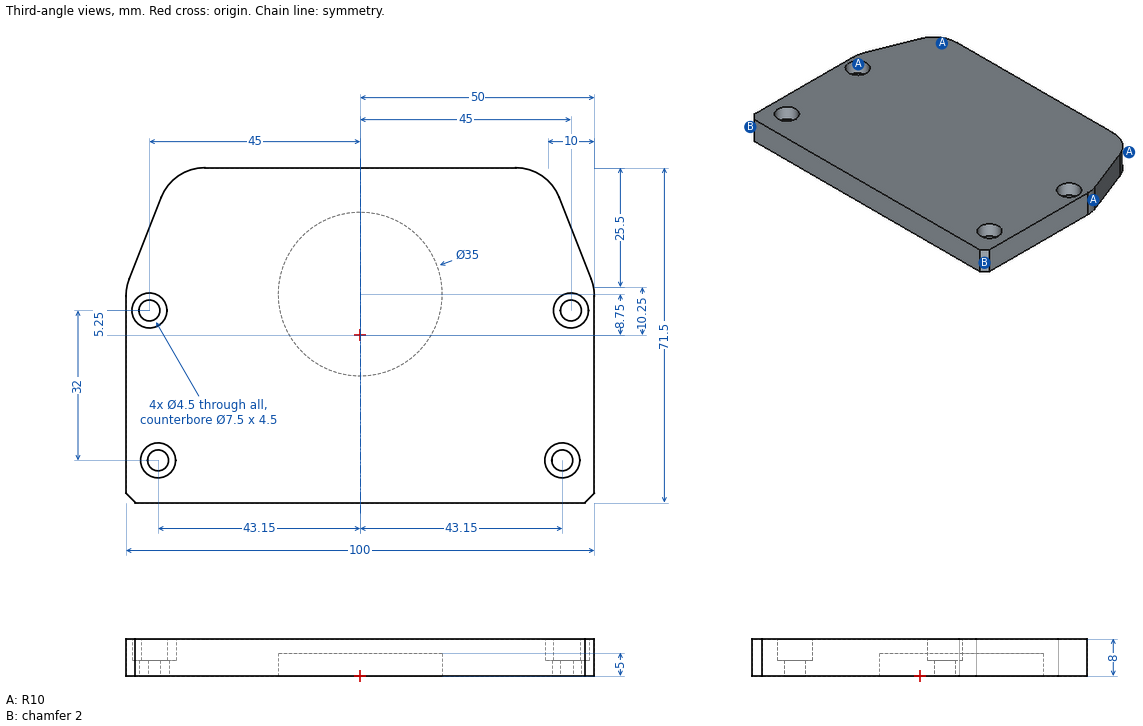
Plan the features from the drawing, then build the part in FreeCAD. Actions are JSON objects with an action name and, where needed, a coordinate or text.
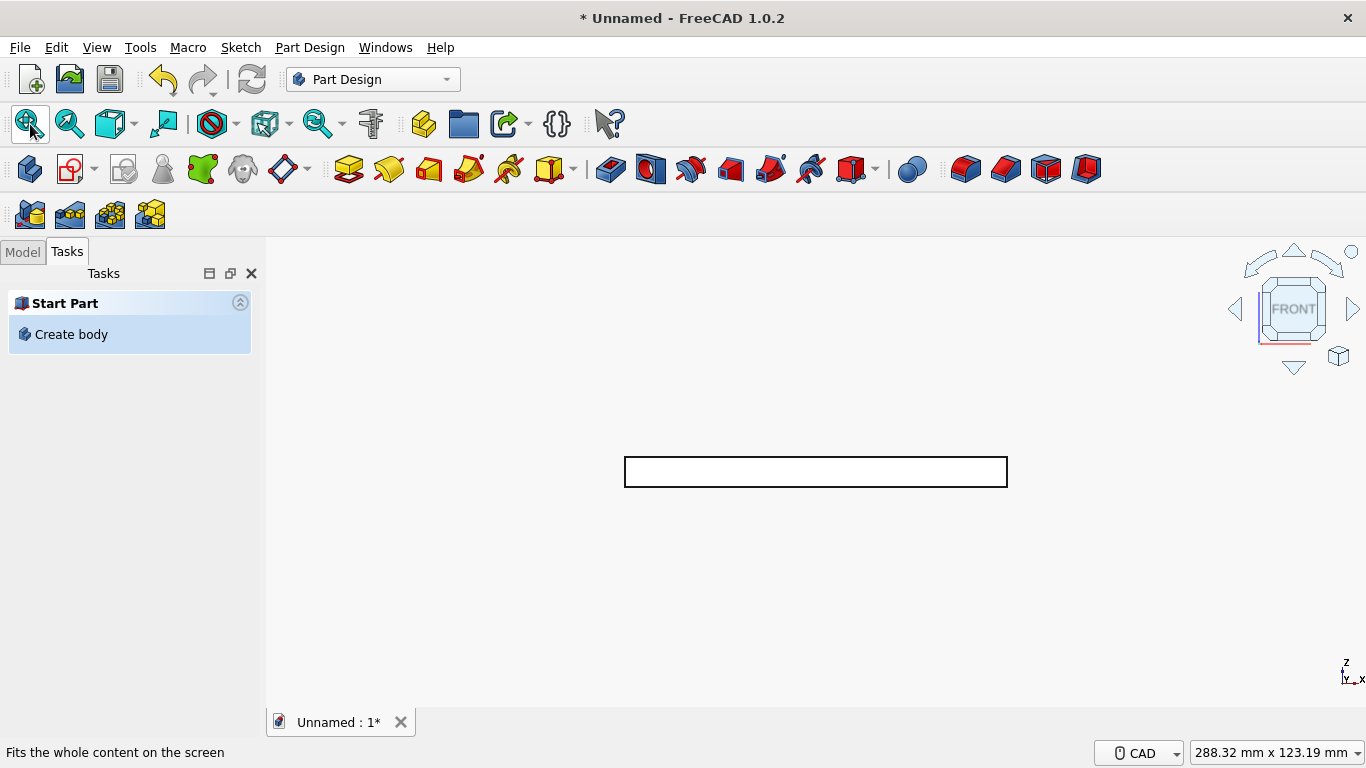
{"action": "key", "text": "3"}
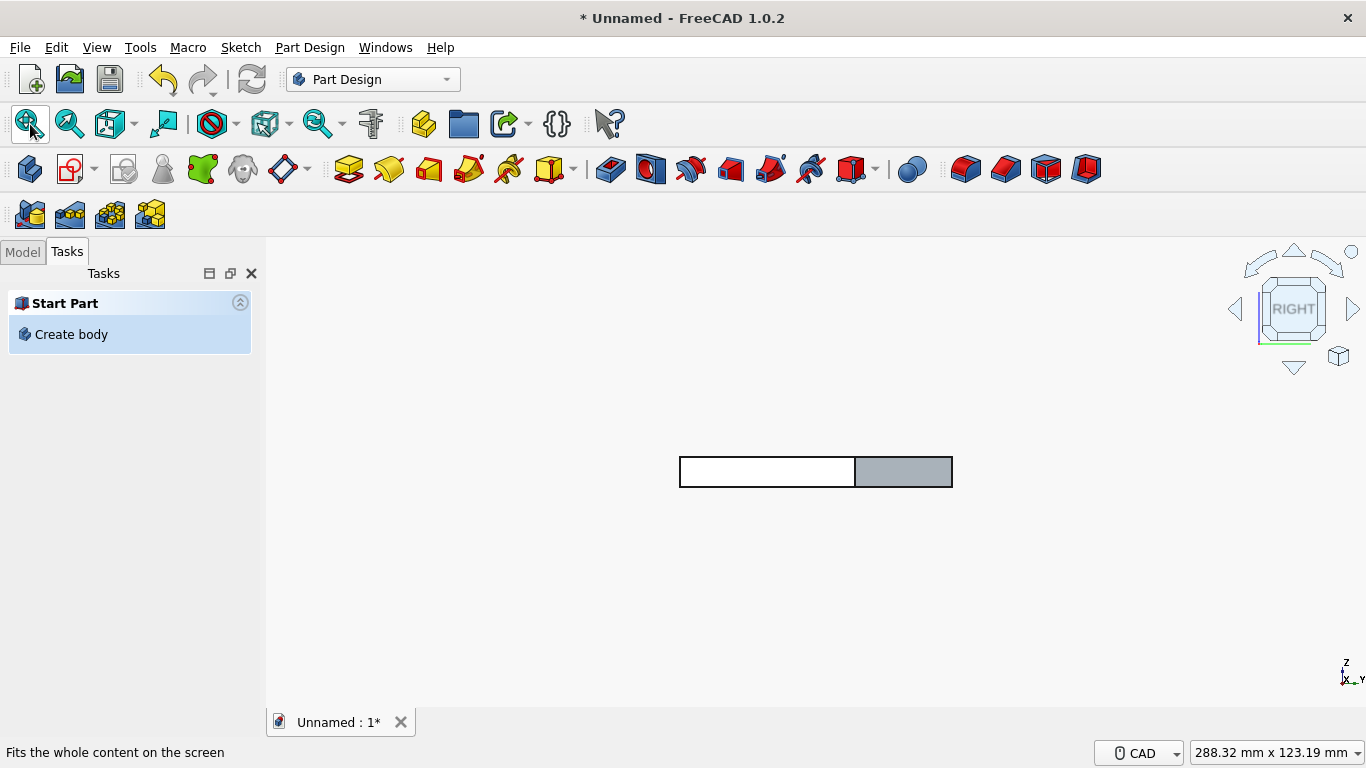
{"action": "left_click", "coordinate": [30, 124]}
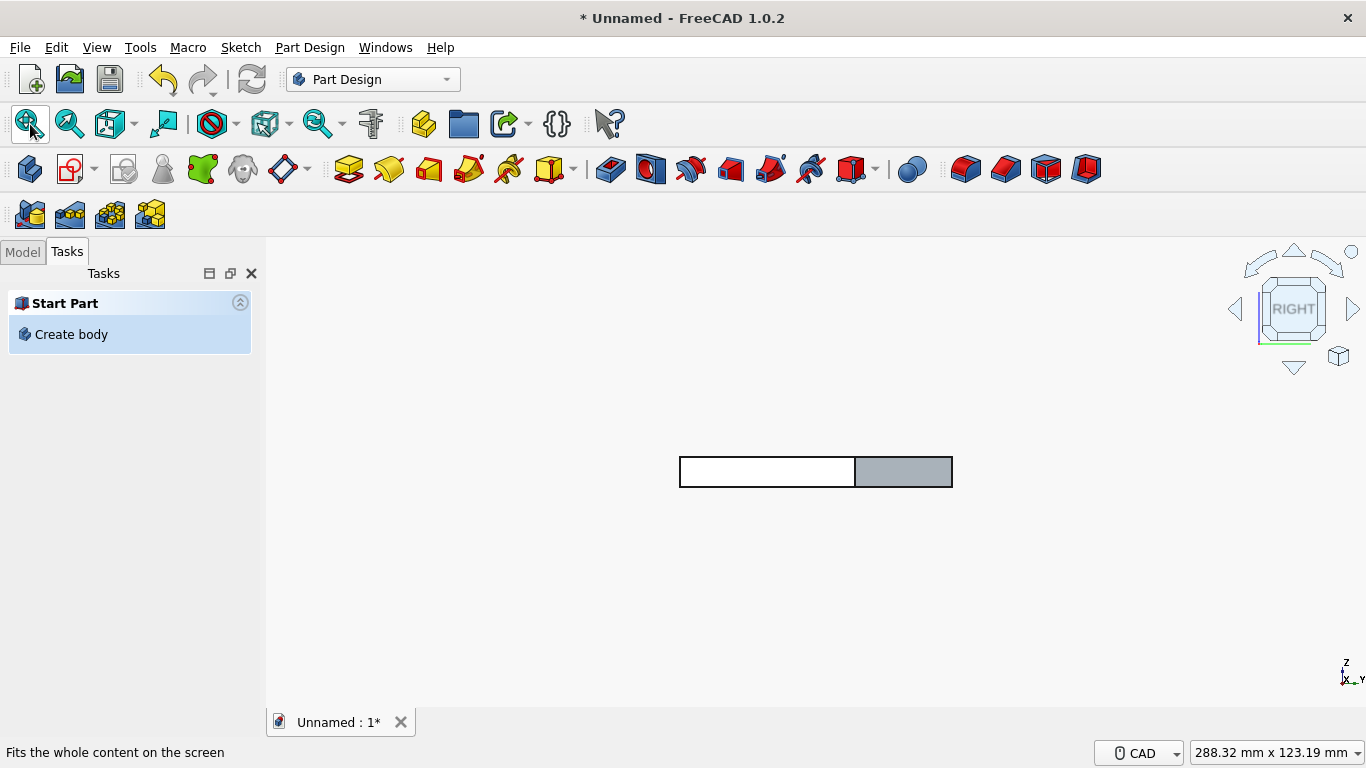
{"action": "left_click", "coordinate": [855, 471]}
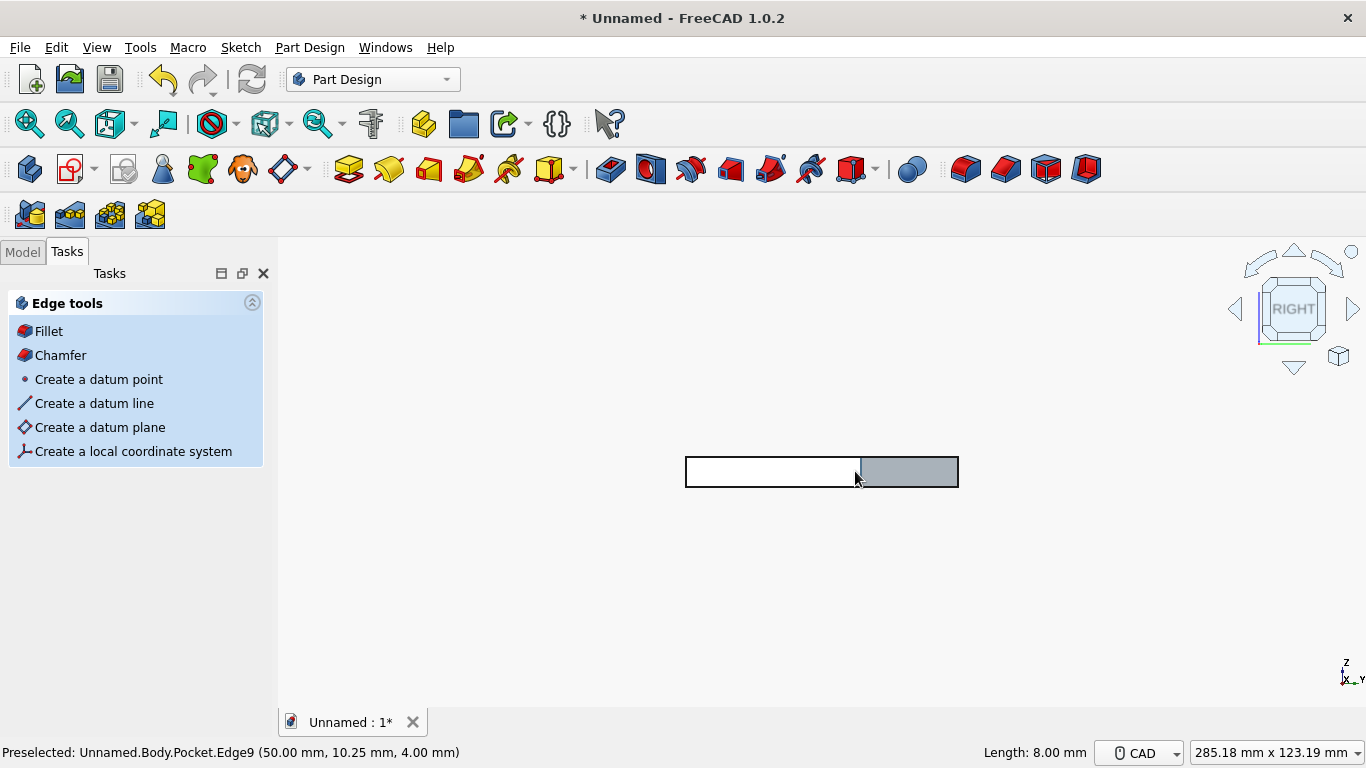
{"action": "key", "text": "5"}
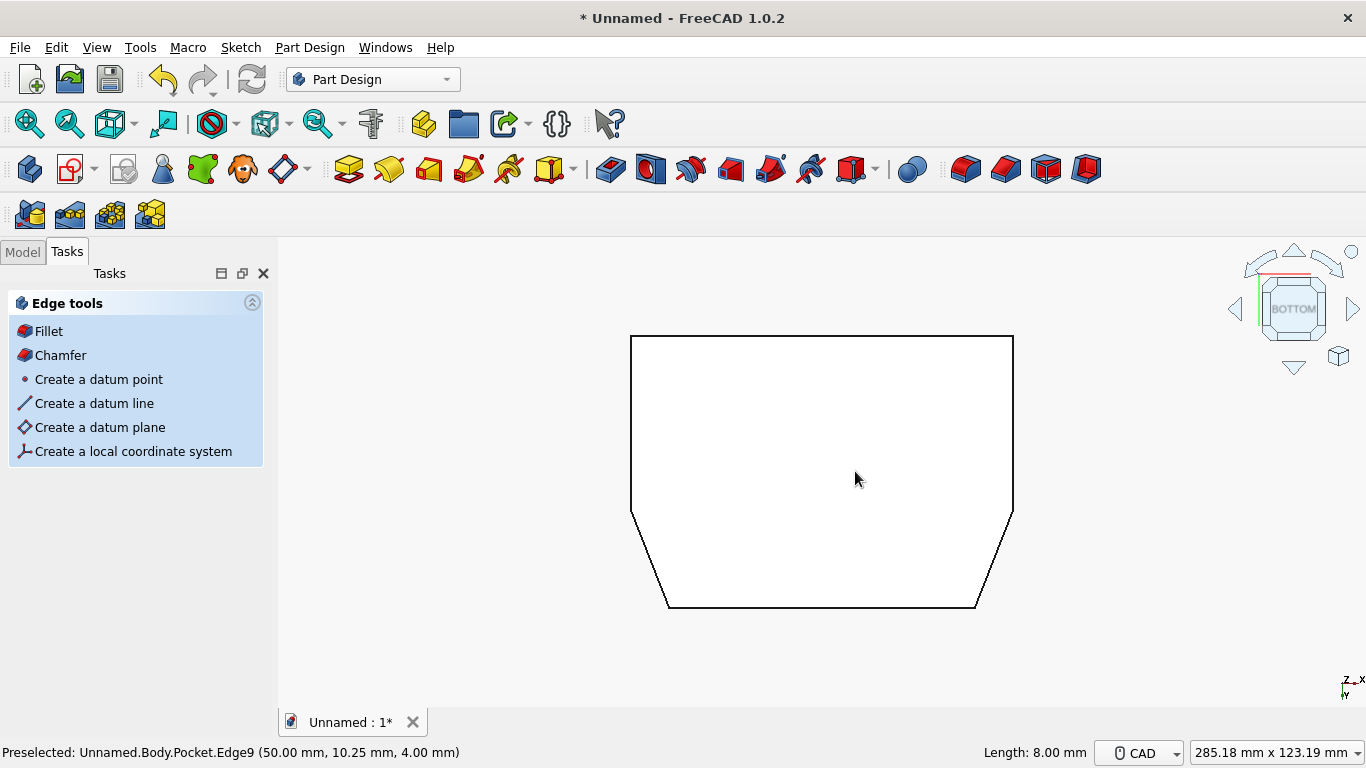
{"action": "key", "text": "4"}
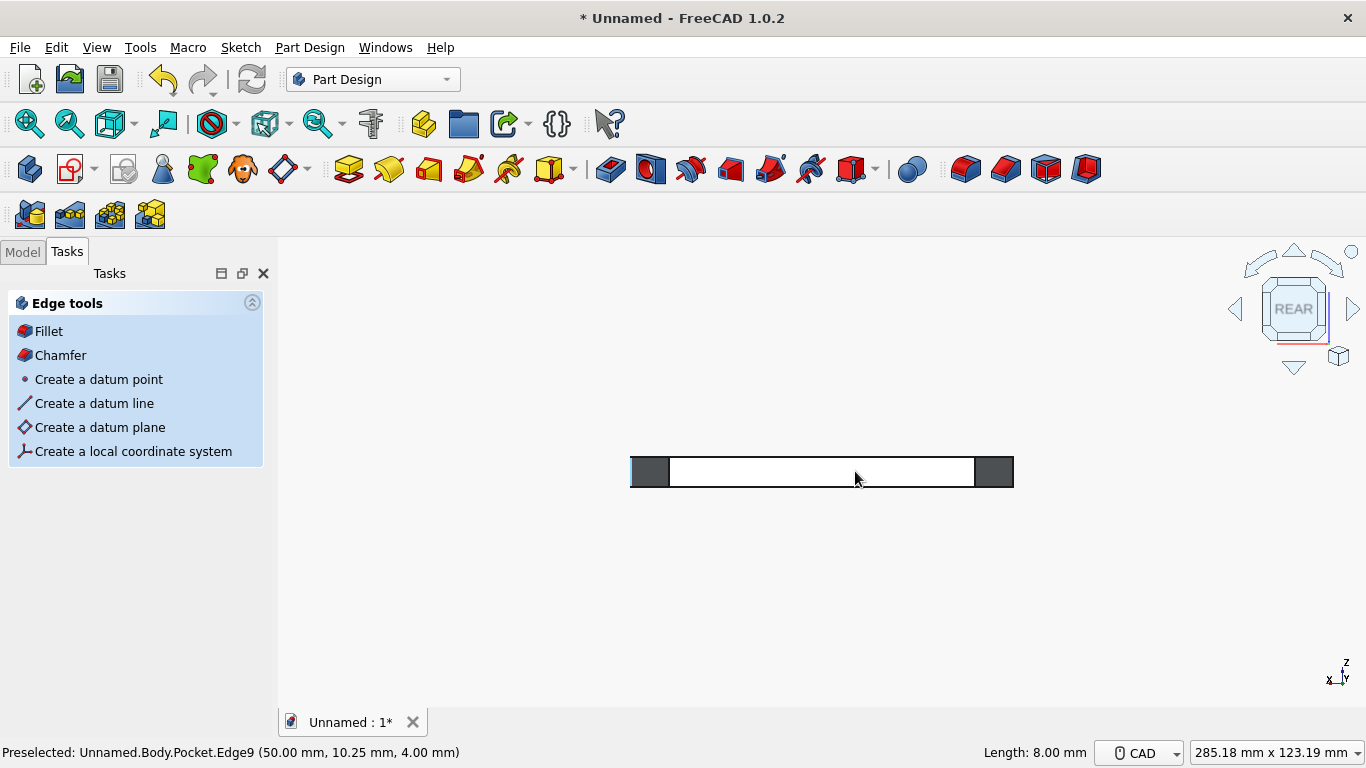
{"action": "left_click", "coordinate": [30, 124]}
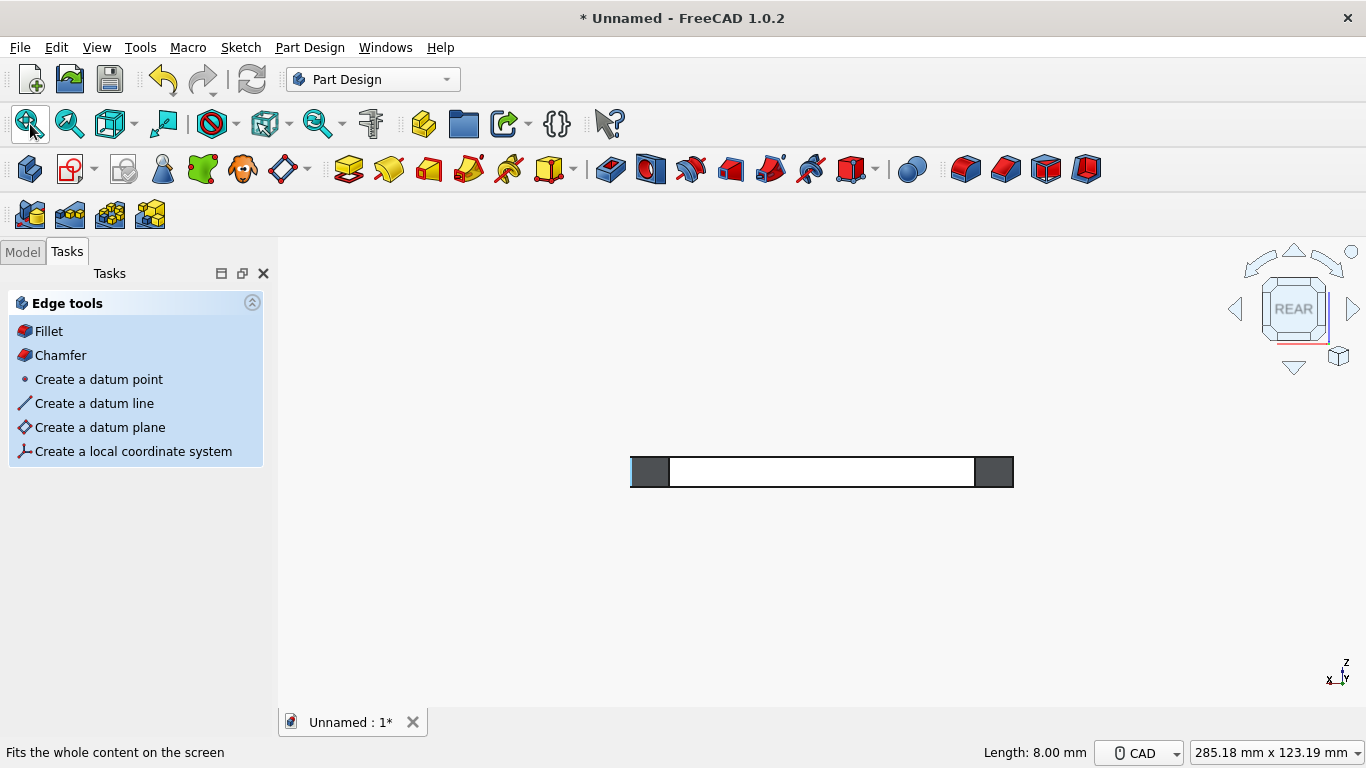
{"action": "left_click", "coordinate": [669, 471], "text": "ctrl"}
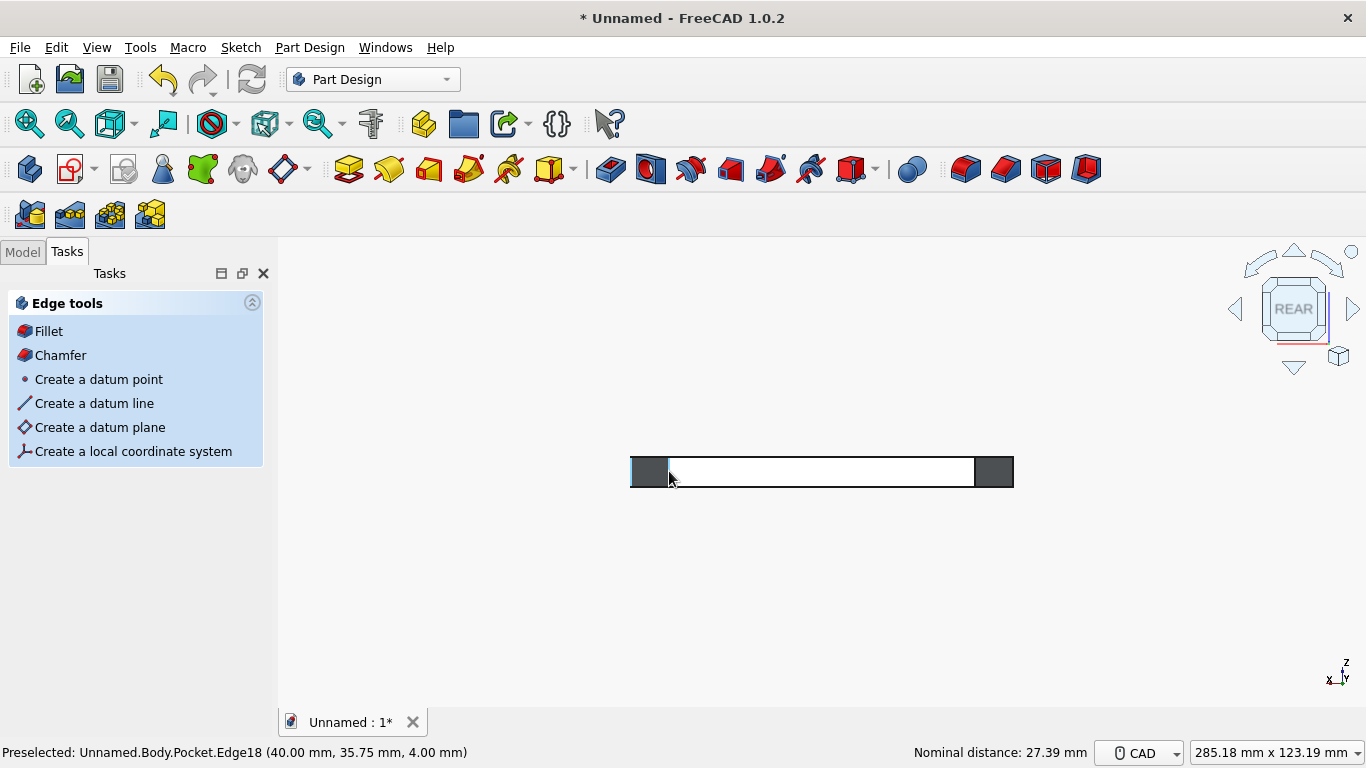
{"action": "left_click", "coordinate": [975, 471], "text": "ctrl"}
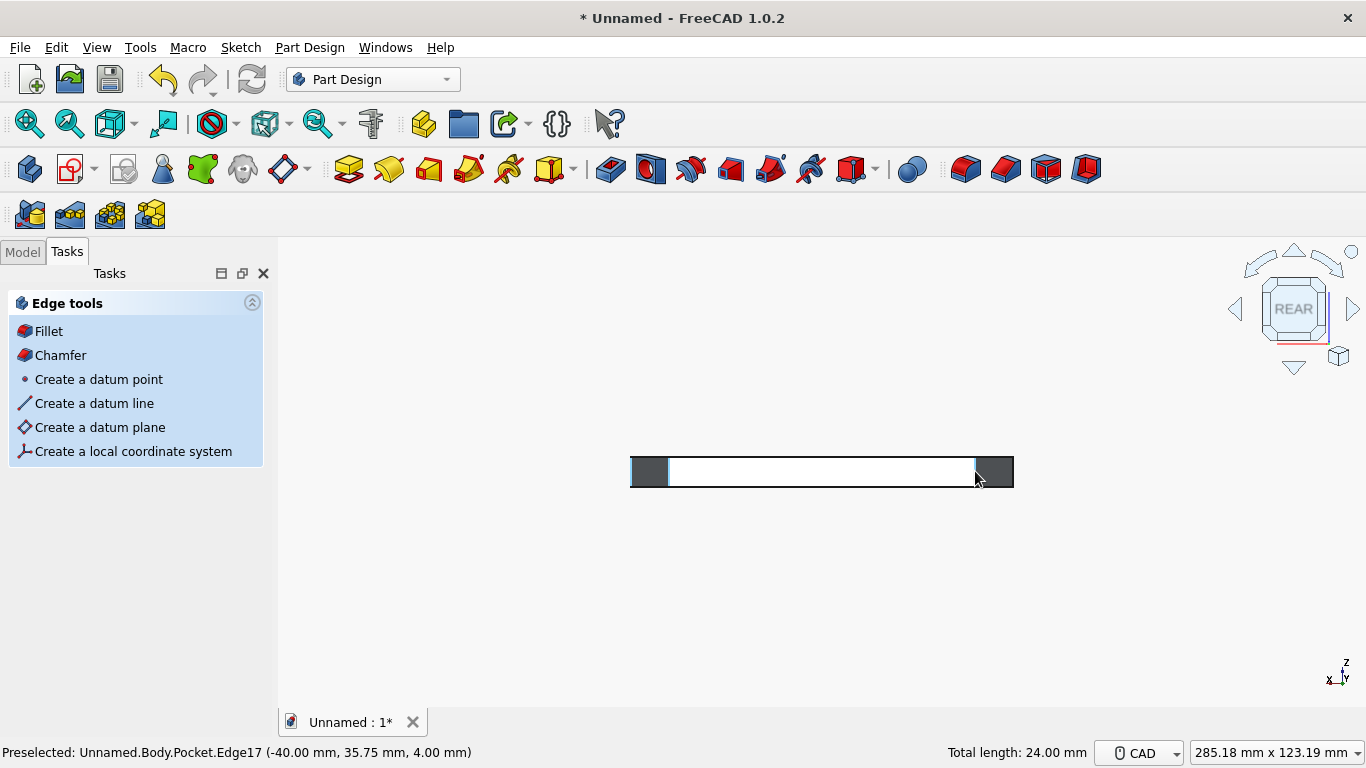
{"action": "key", "text": "6"}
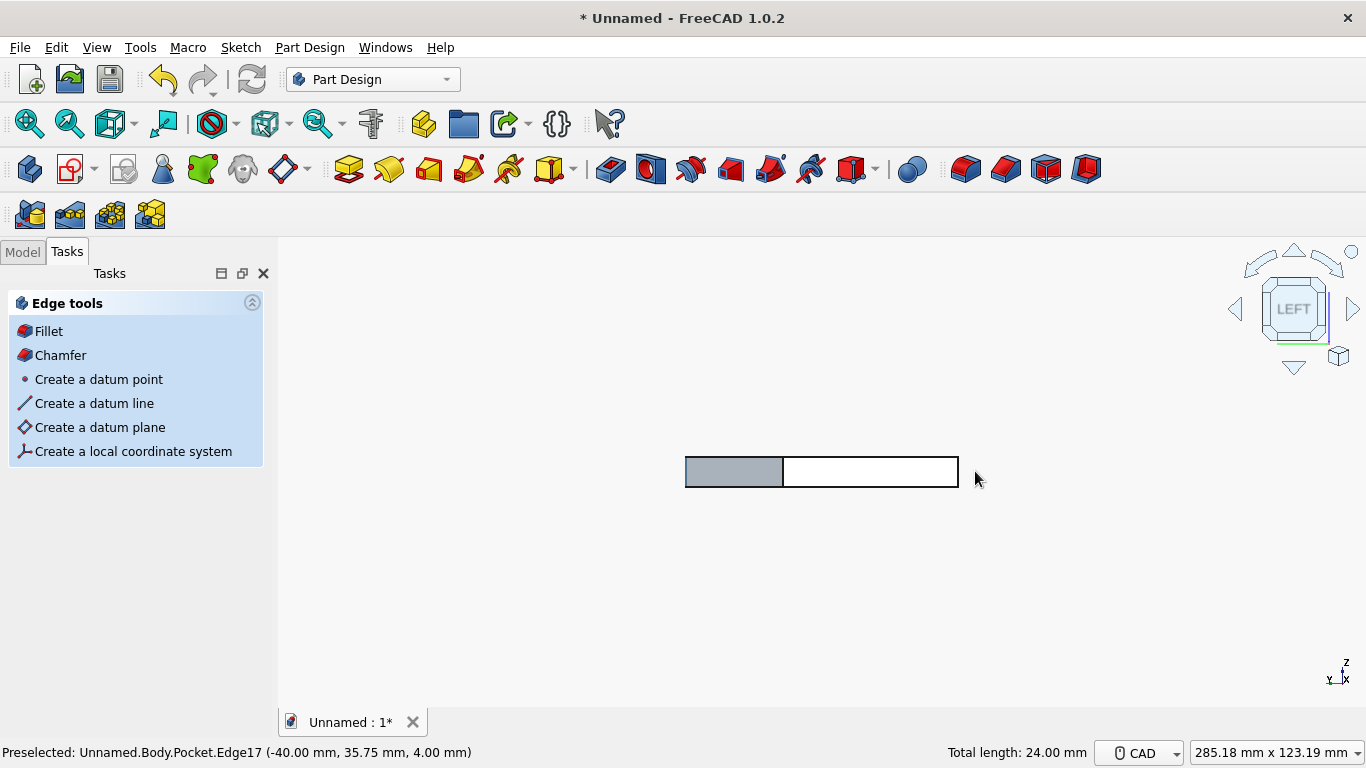
{"action": "left_click", "coordinate": [30, 124]}